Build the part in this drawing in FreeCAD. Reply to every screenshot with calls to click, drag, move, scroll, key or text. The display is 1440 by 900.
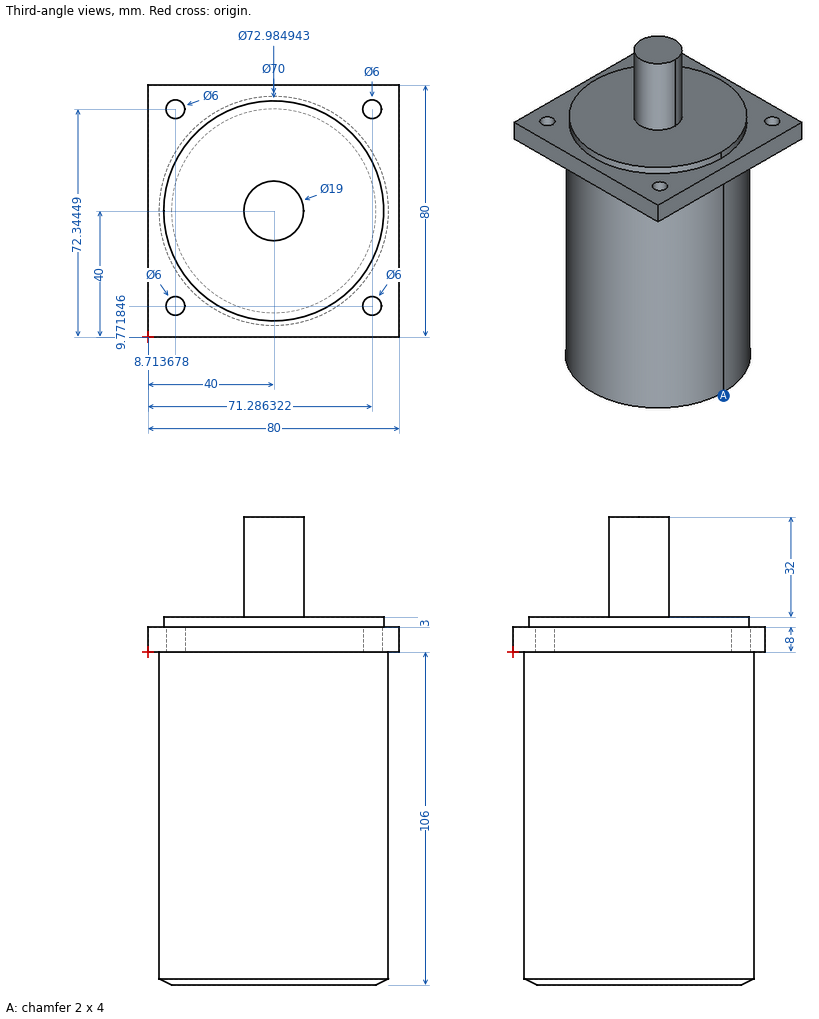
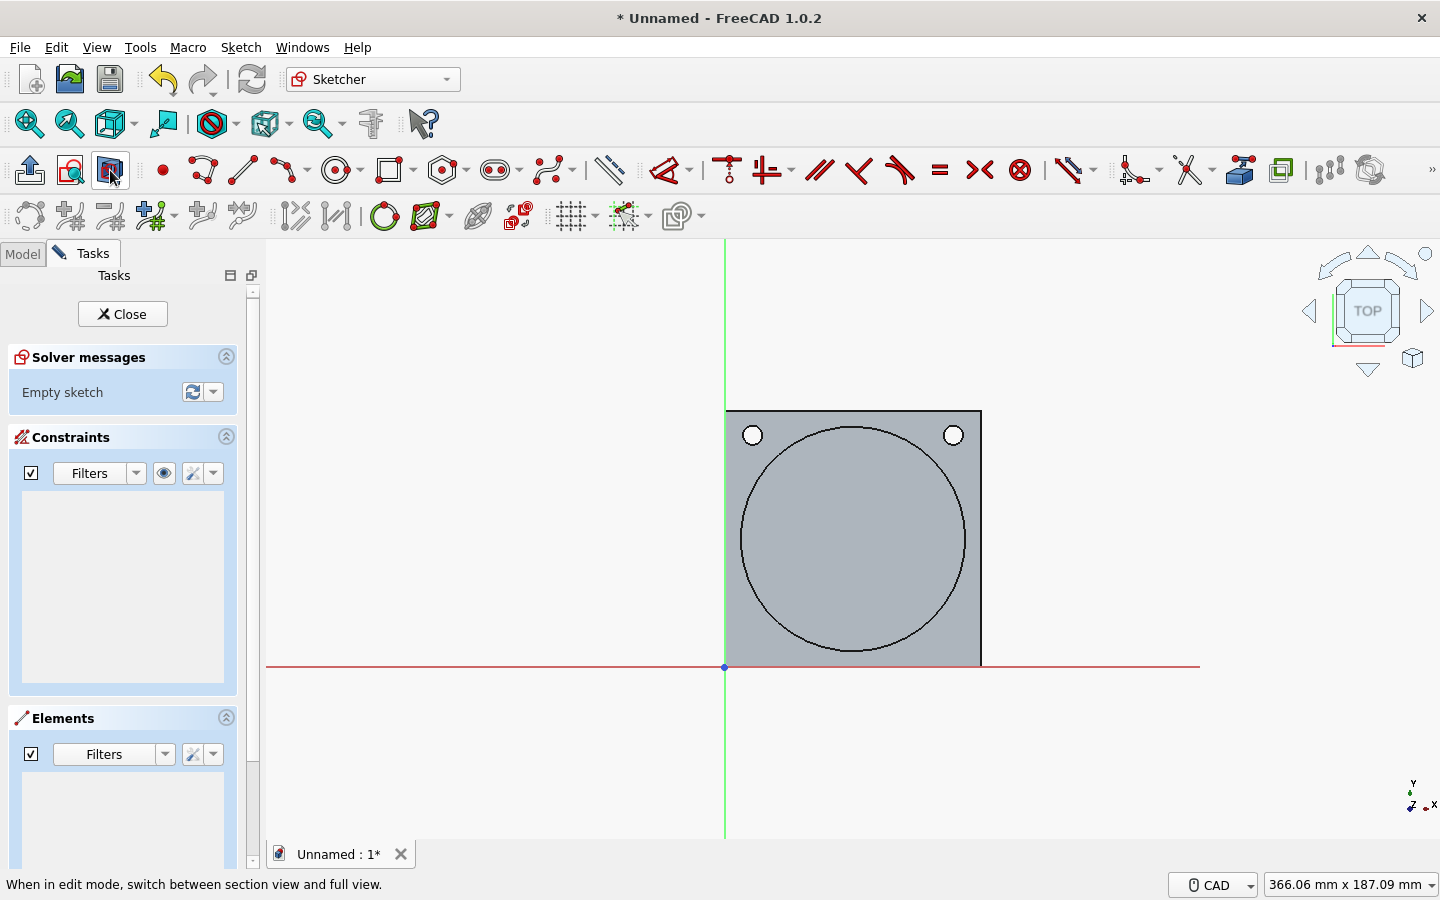
scroll(962, 641, up, 15)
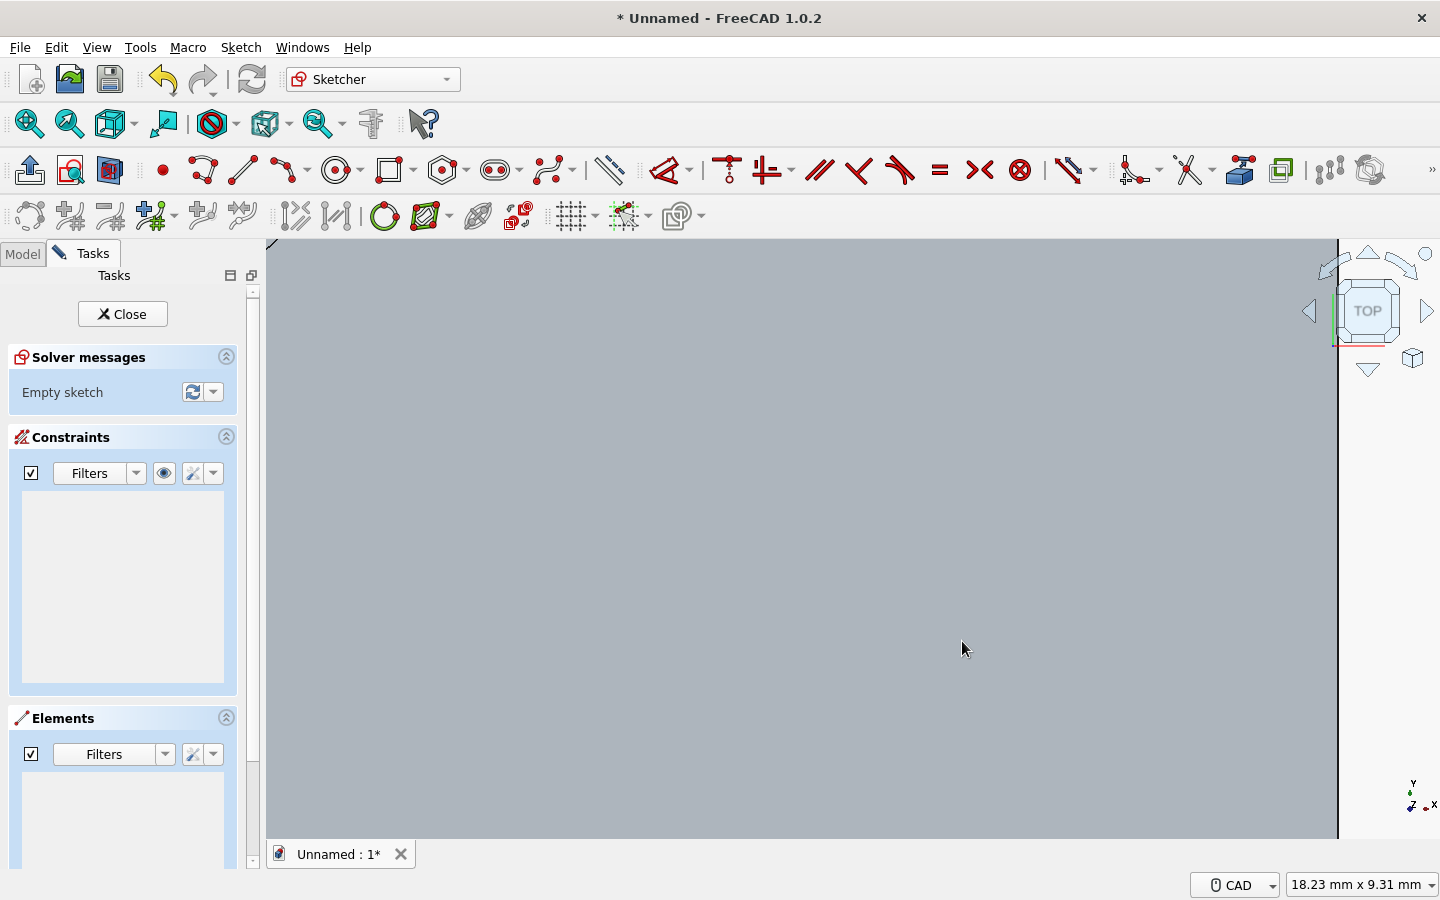
click(336, 170)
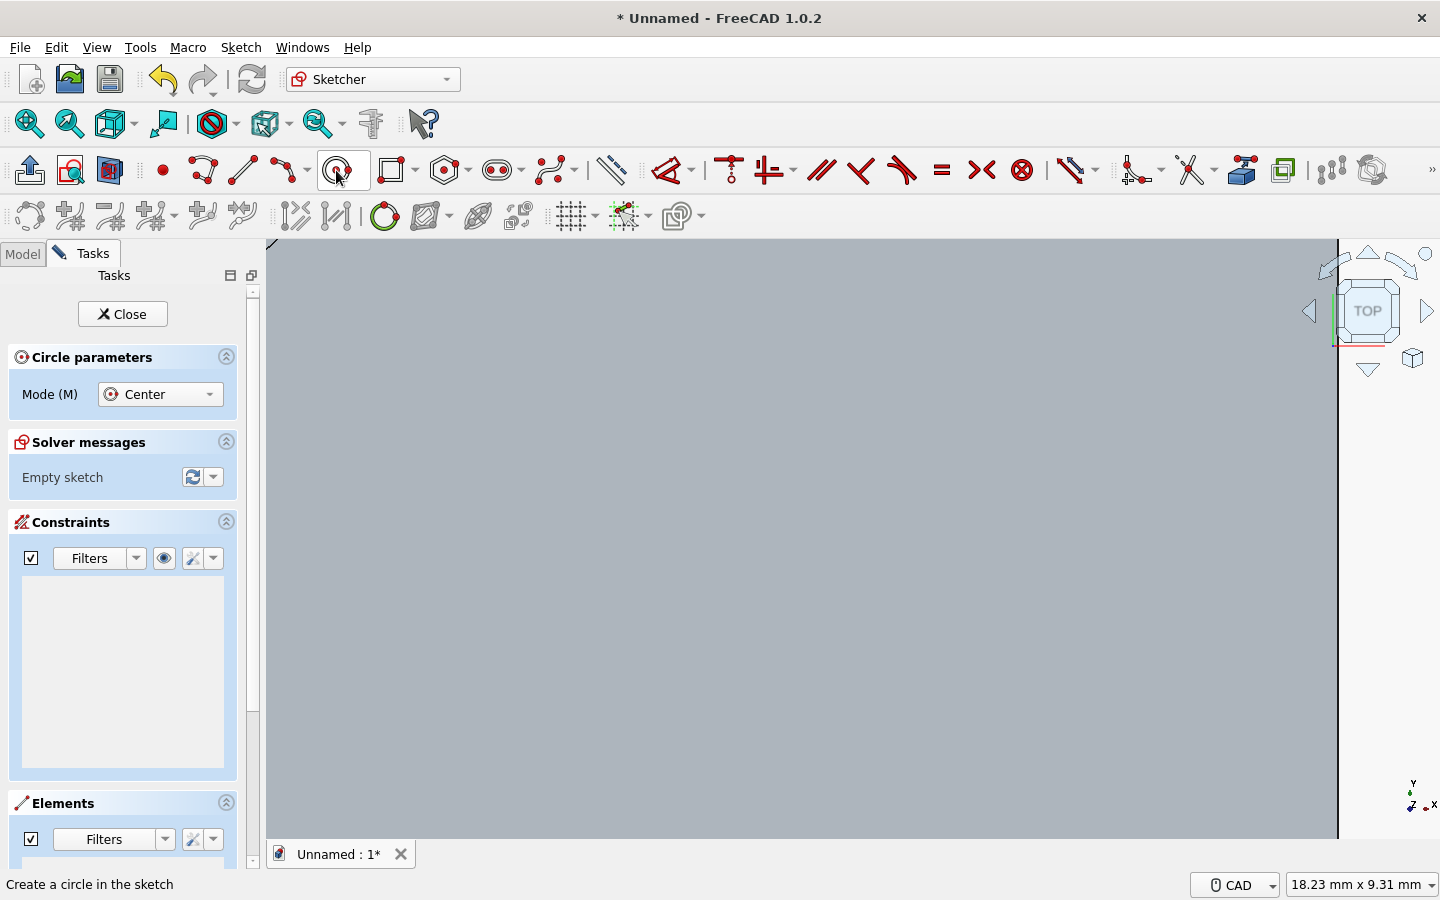
click(777, 527)
move(913, 390)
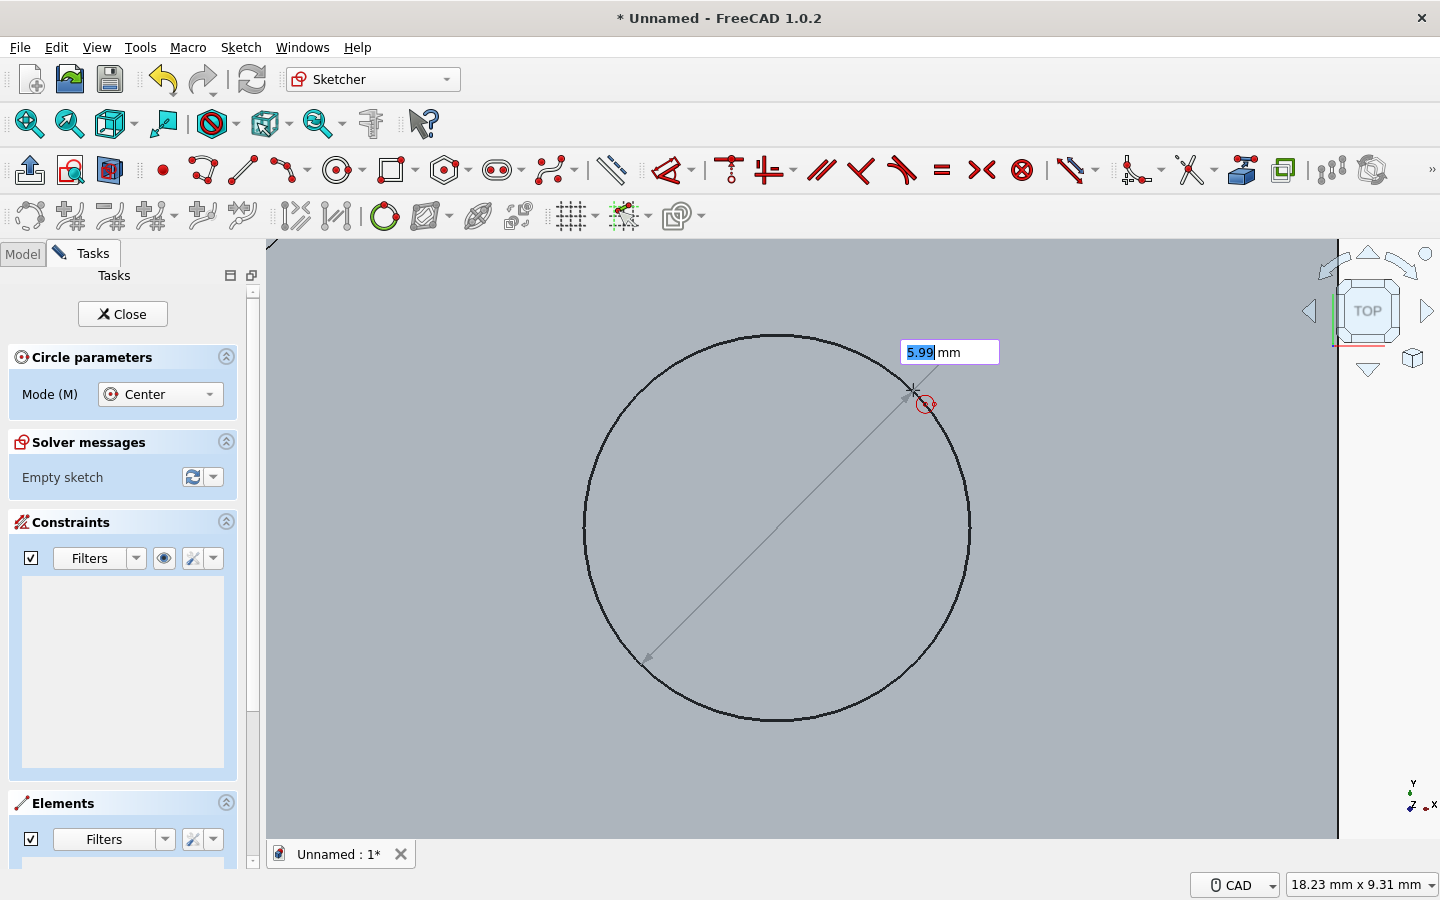
text(6)
key(Return)
key(Escape)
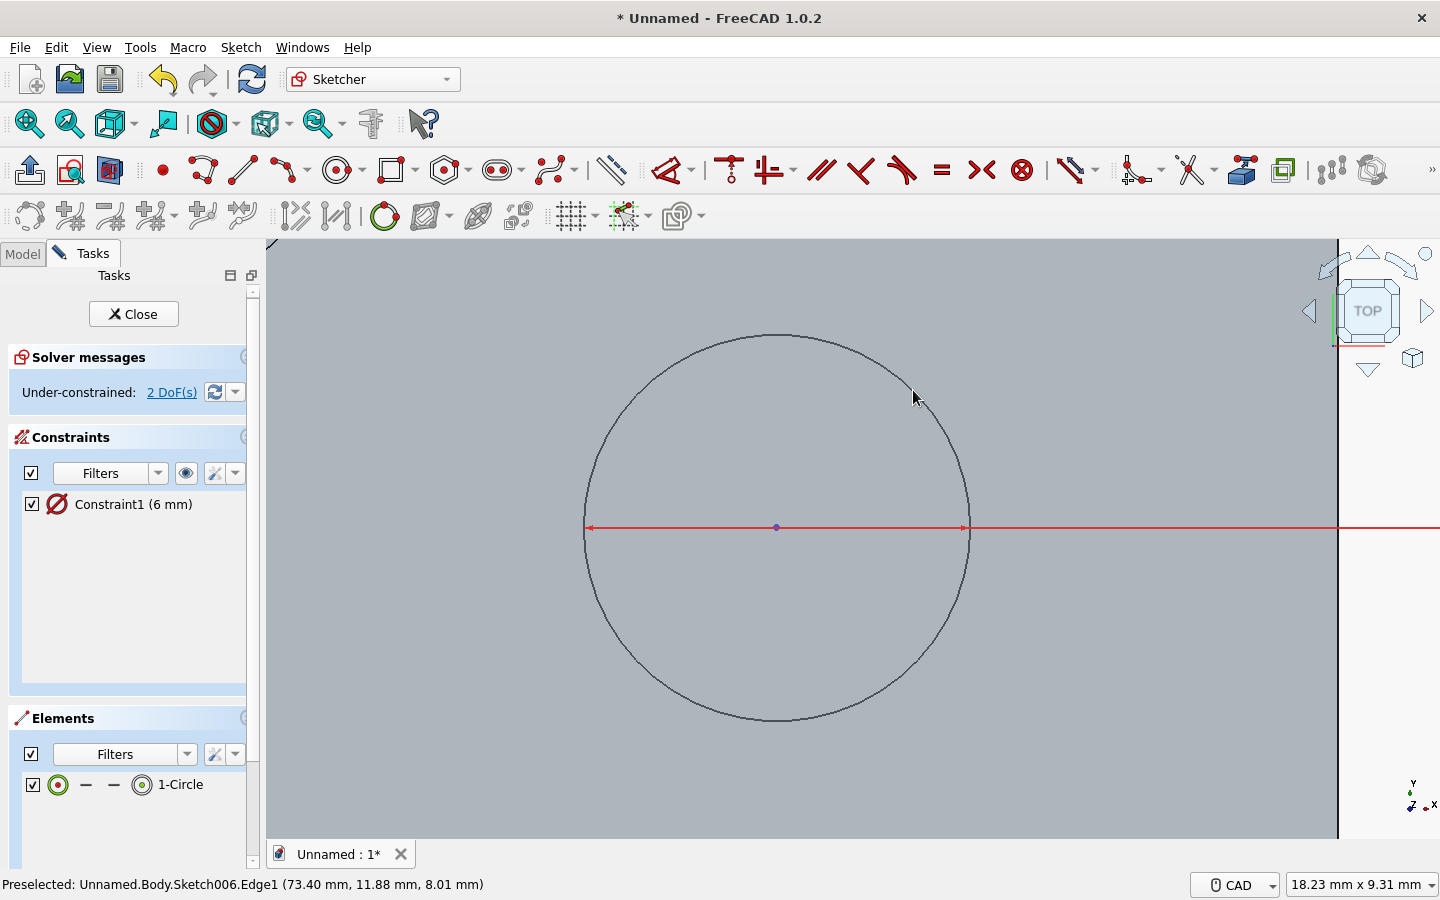
click(666, 170)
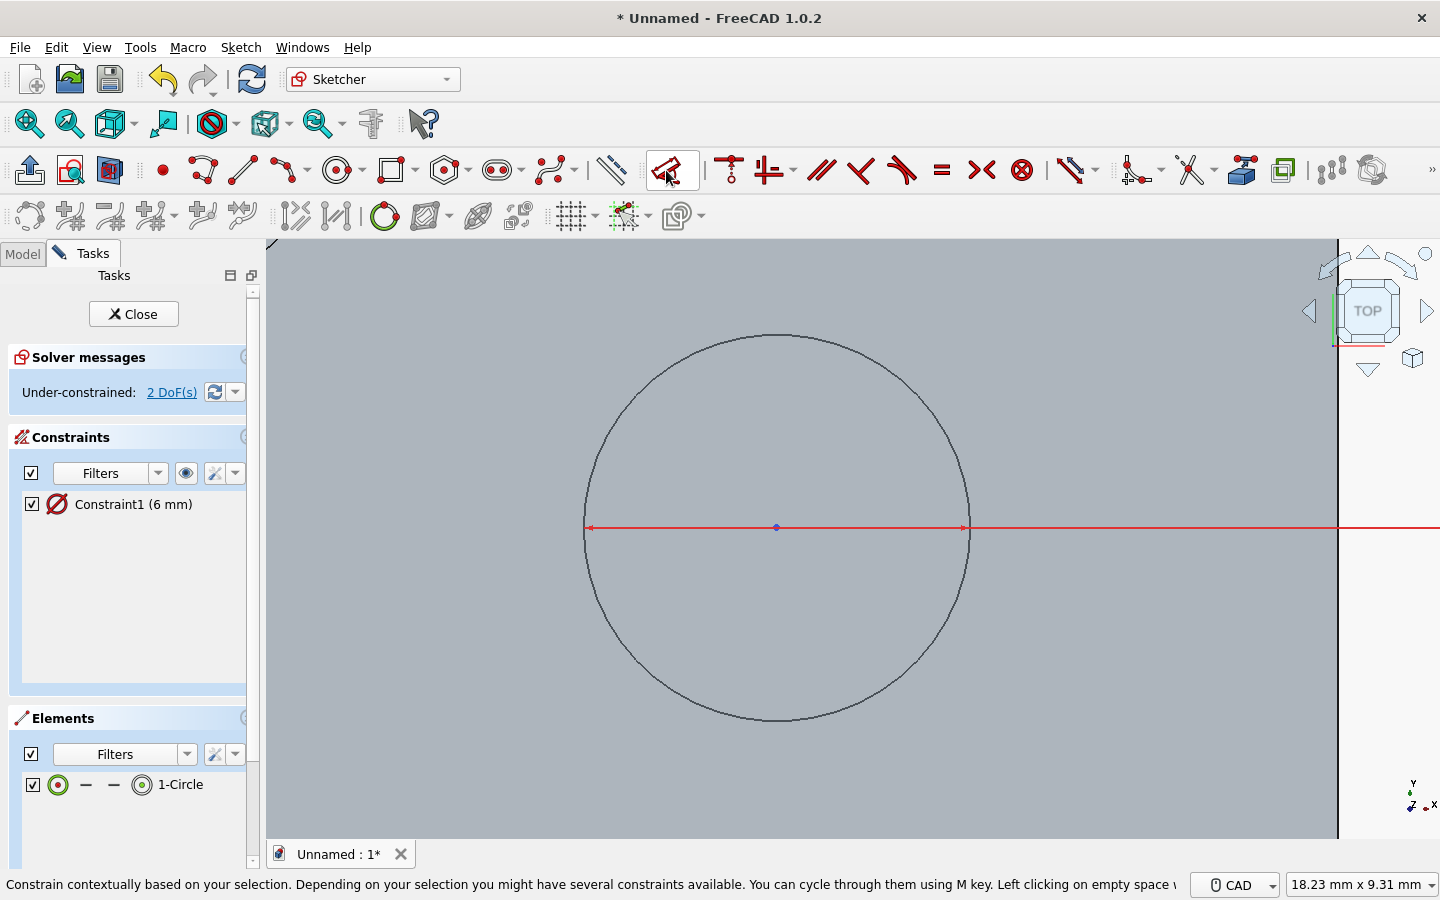
click(777, 528)
click(811, 669)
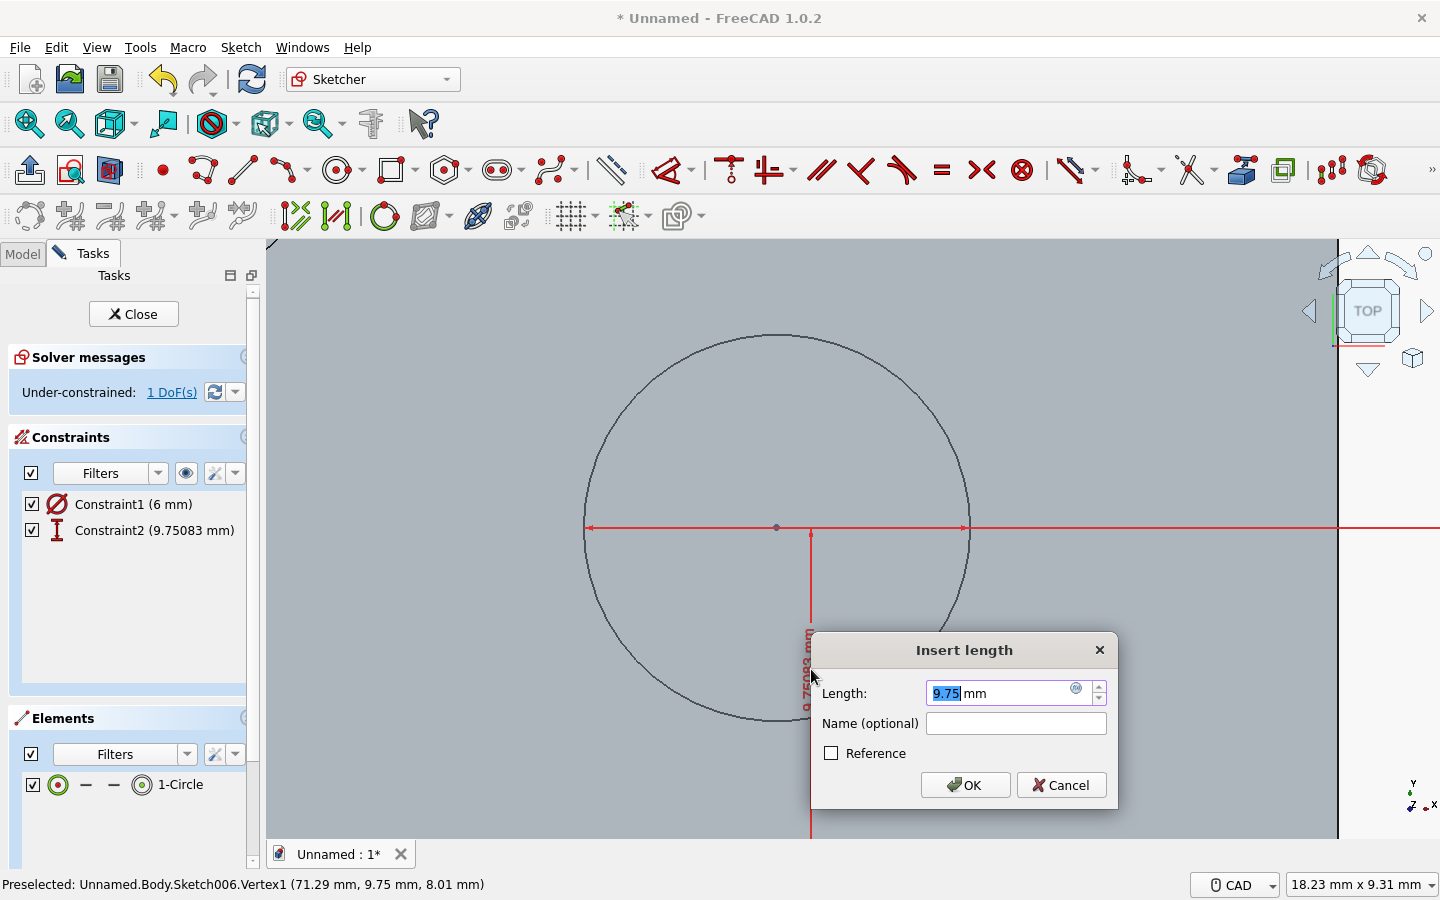
text(9.771846)
key(Return)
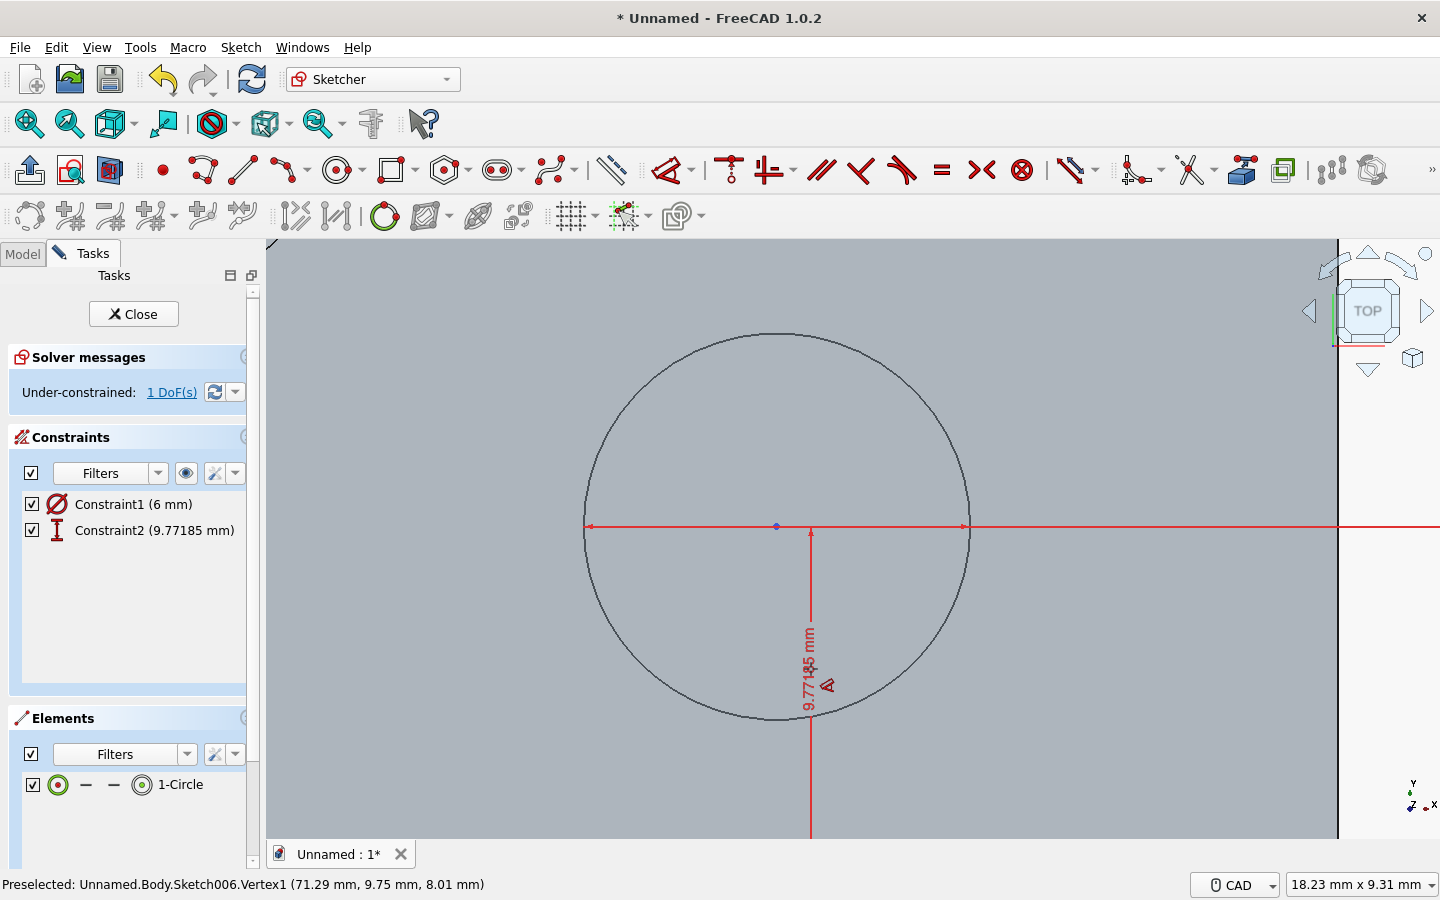
click(777, 527)
click(535, 493)